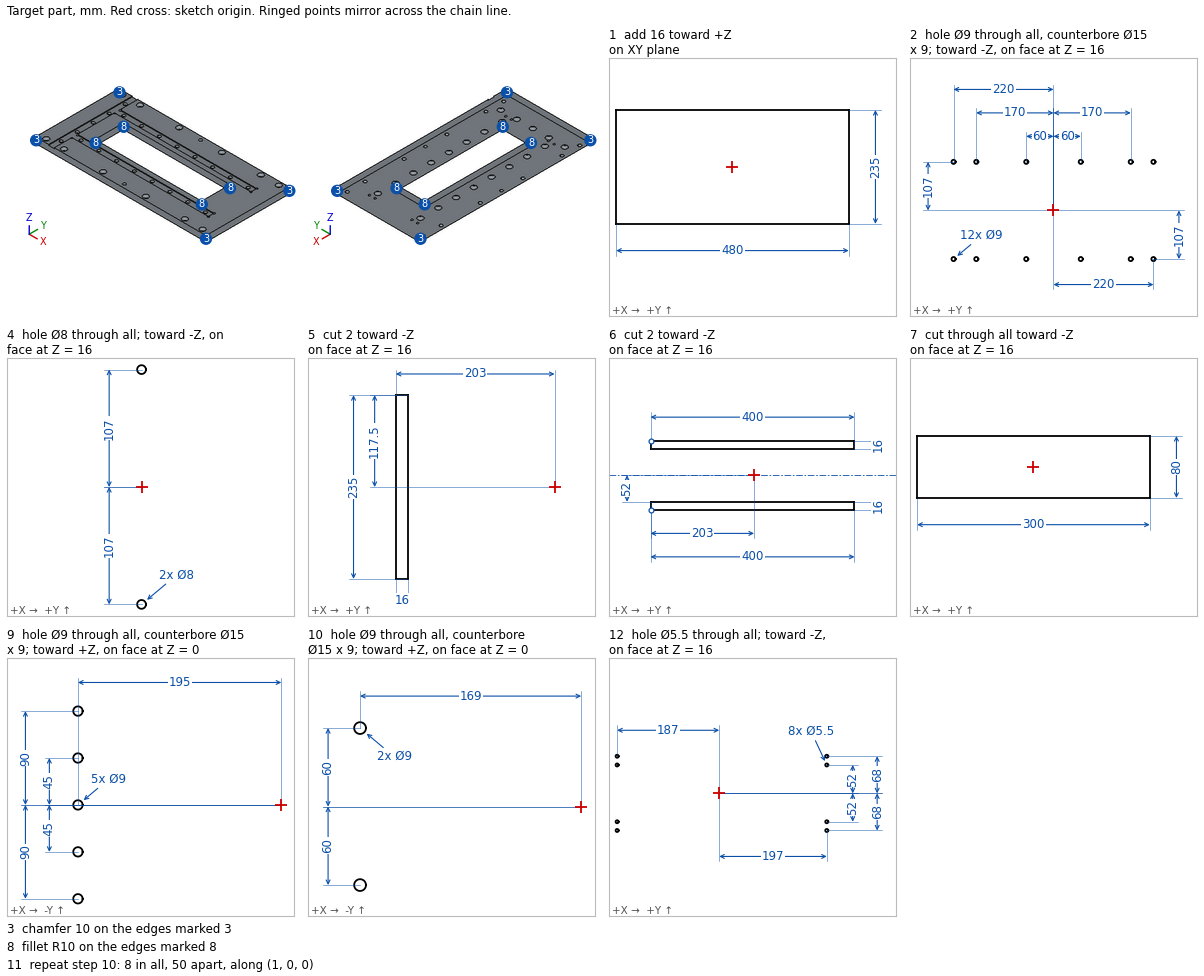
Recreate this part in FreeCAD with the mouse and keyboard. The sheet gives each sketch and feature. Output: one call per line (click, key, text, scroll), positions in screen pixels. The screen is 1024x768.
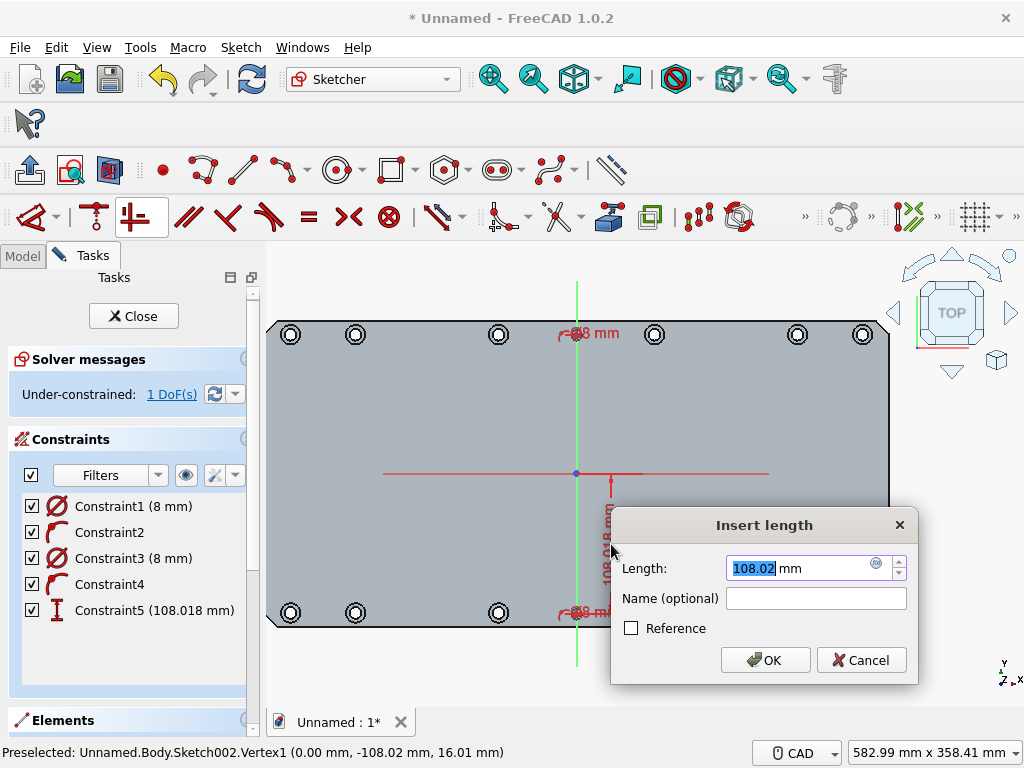
text(107)
key(Return)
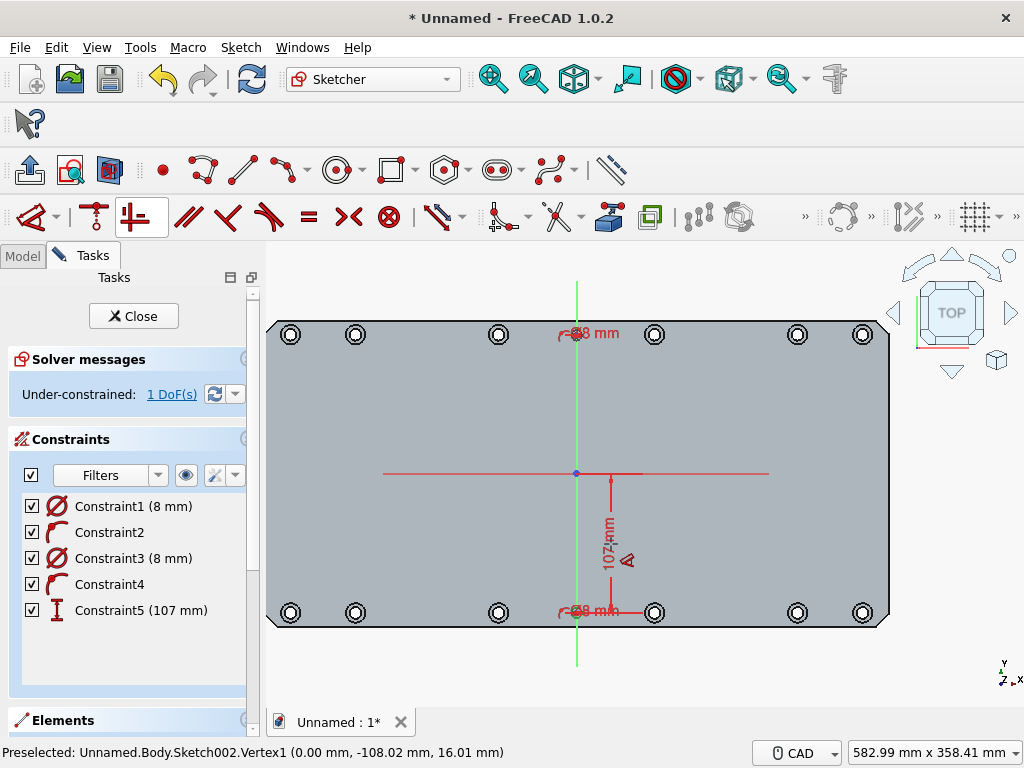
click(577, 335)
click(611, 405)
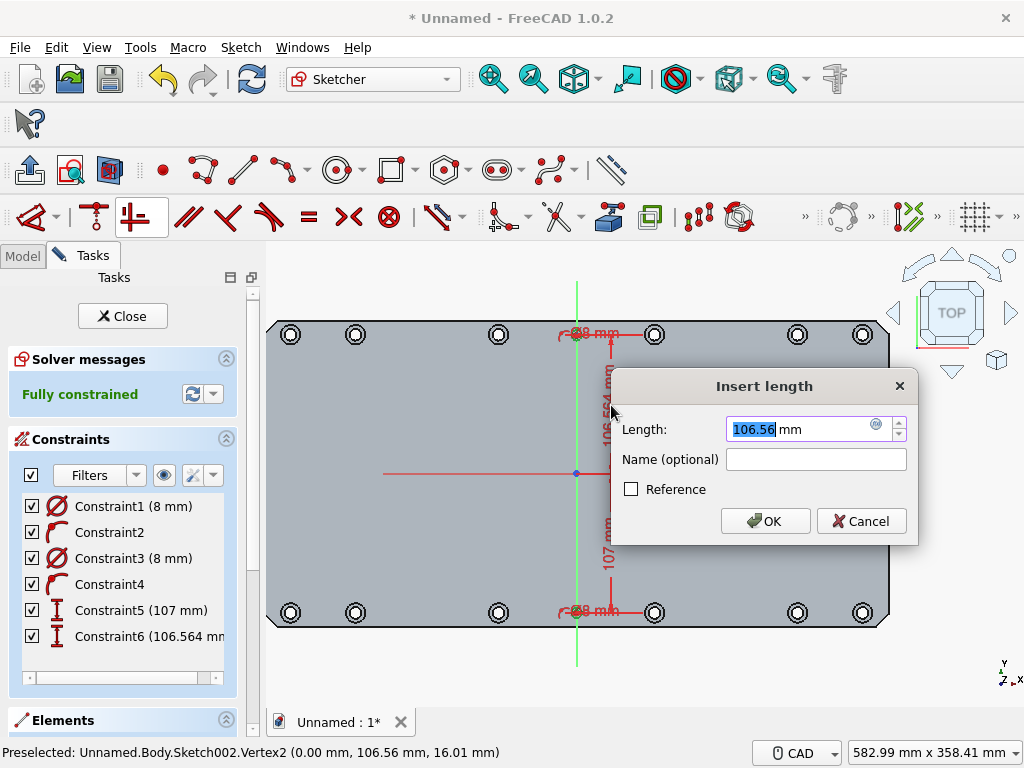
text(107)
key(Return)
key(Escape)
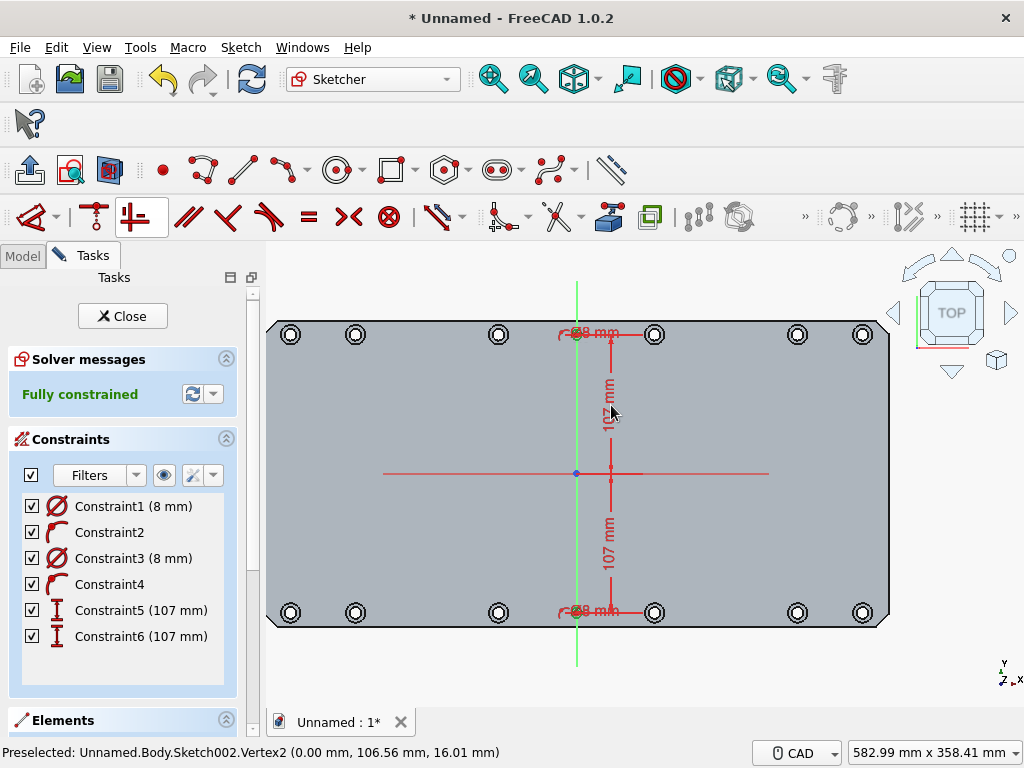
click(123, 316)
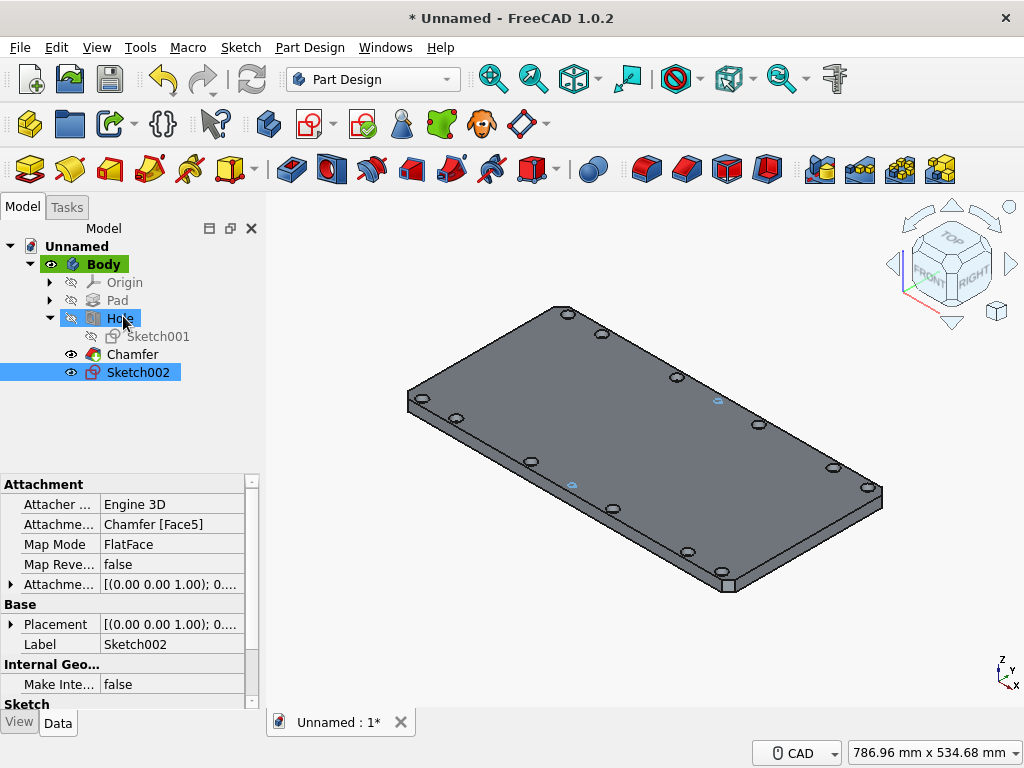
click(332, 170)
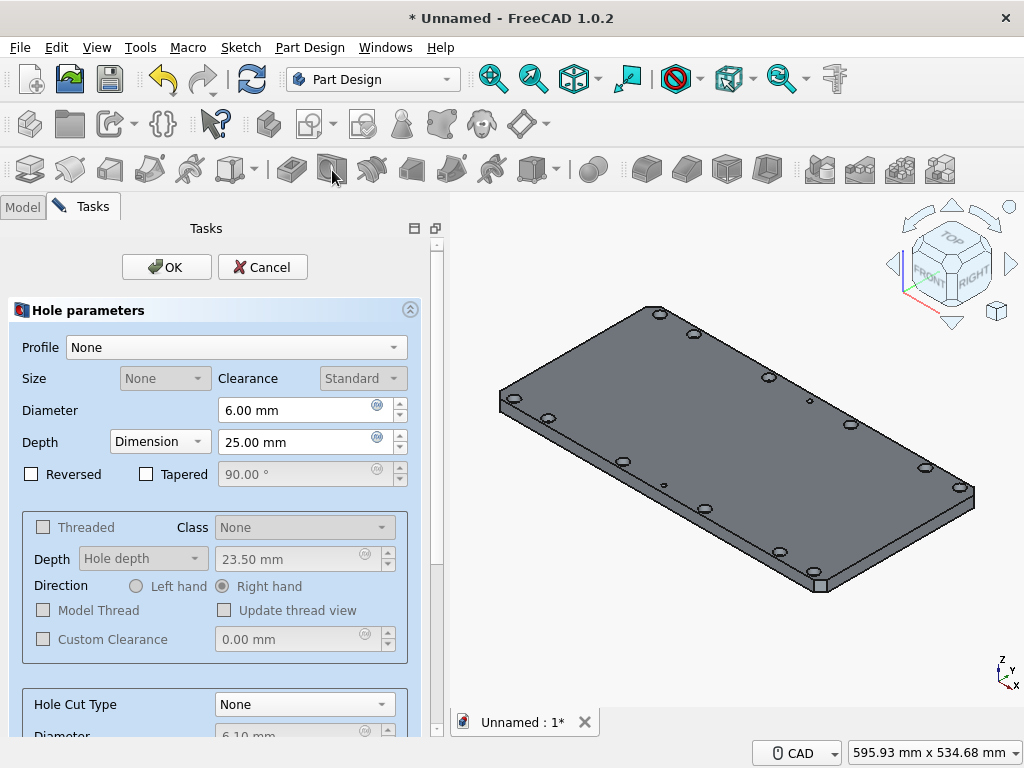
triple_click(305, 410)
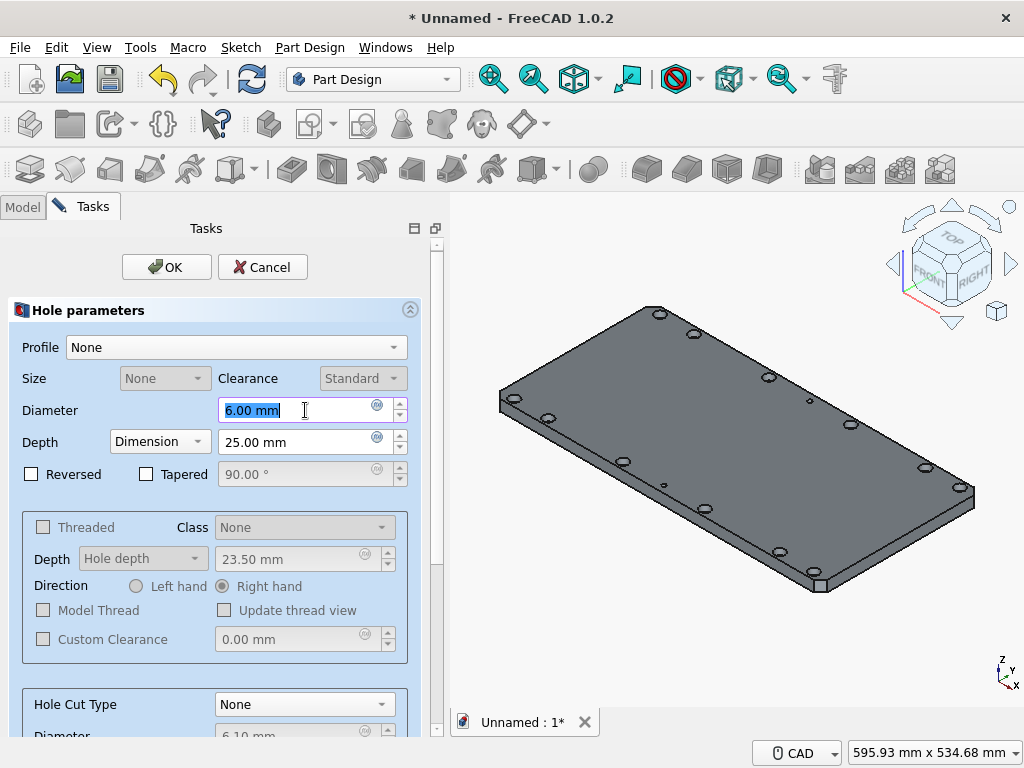
text(8)
key(Tab)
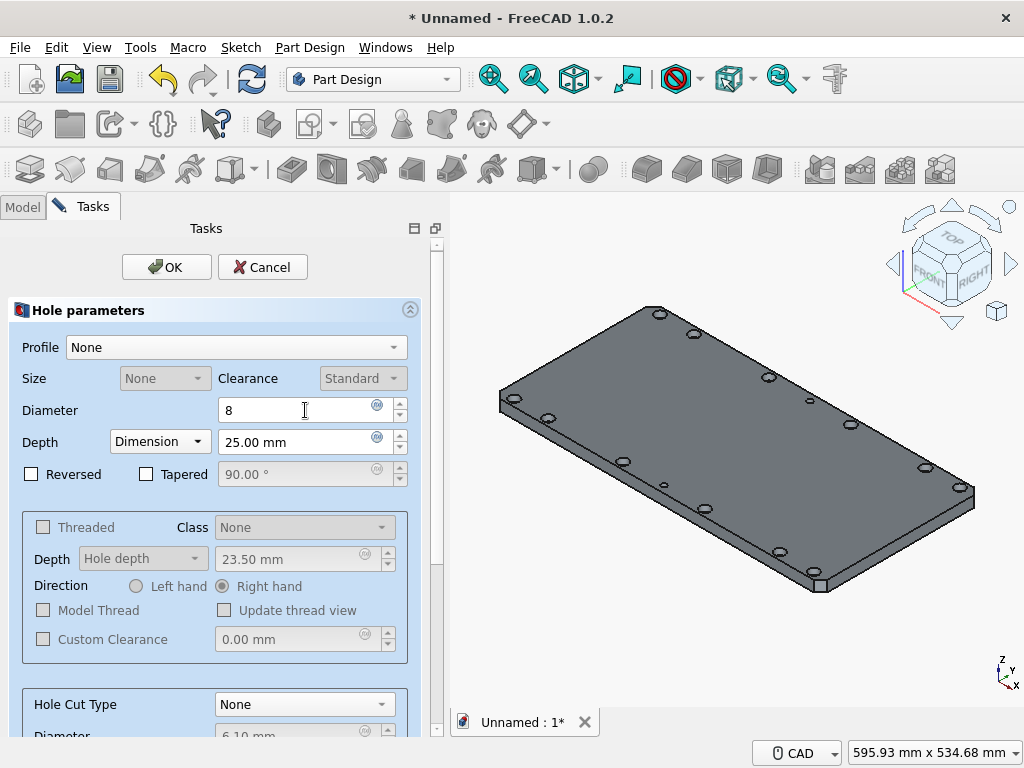
click(161, 442)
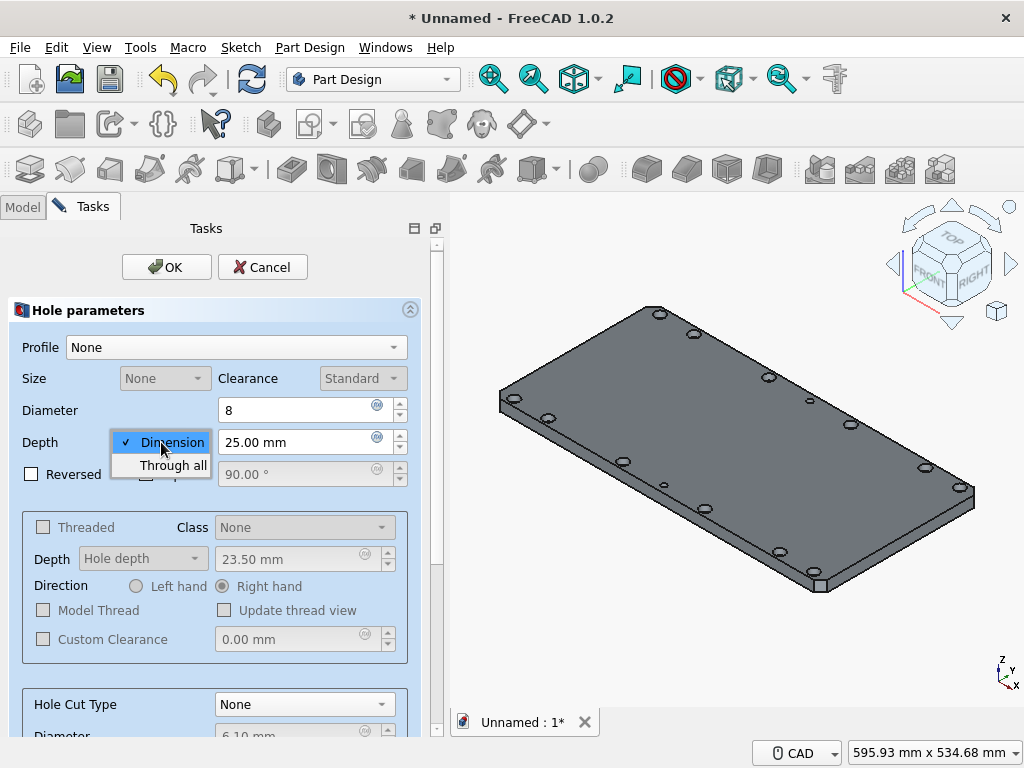
click(160, 466)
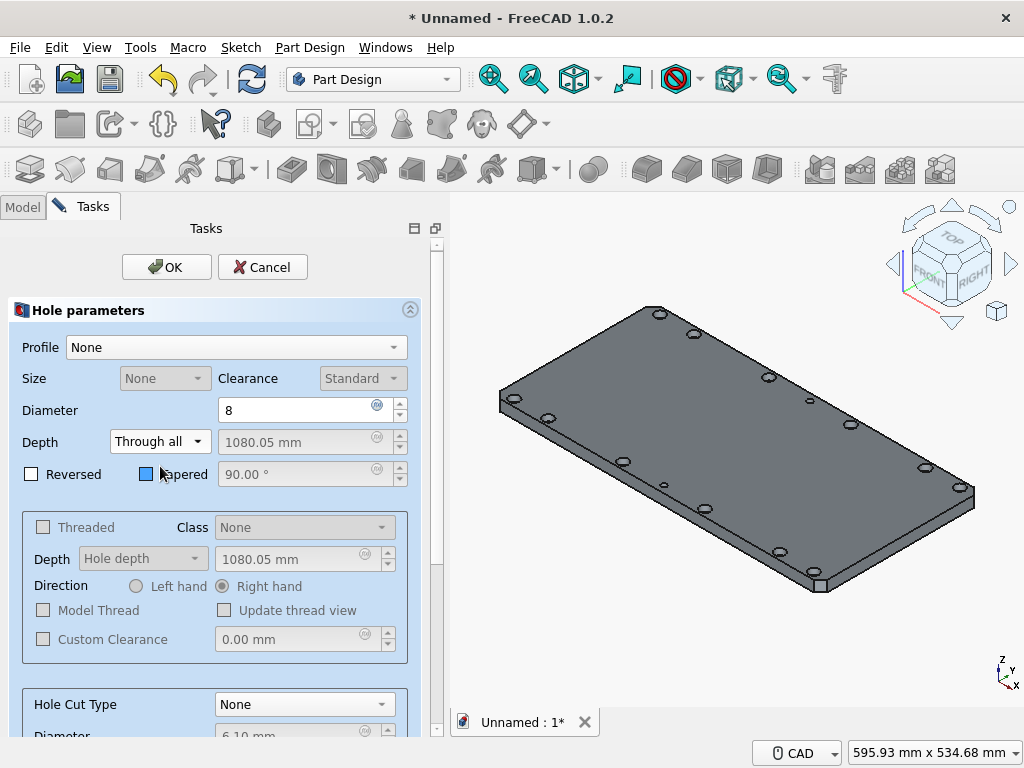
click(167, 267)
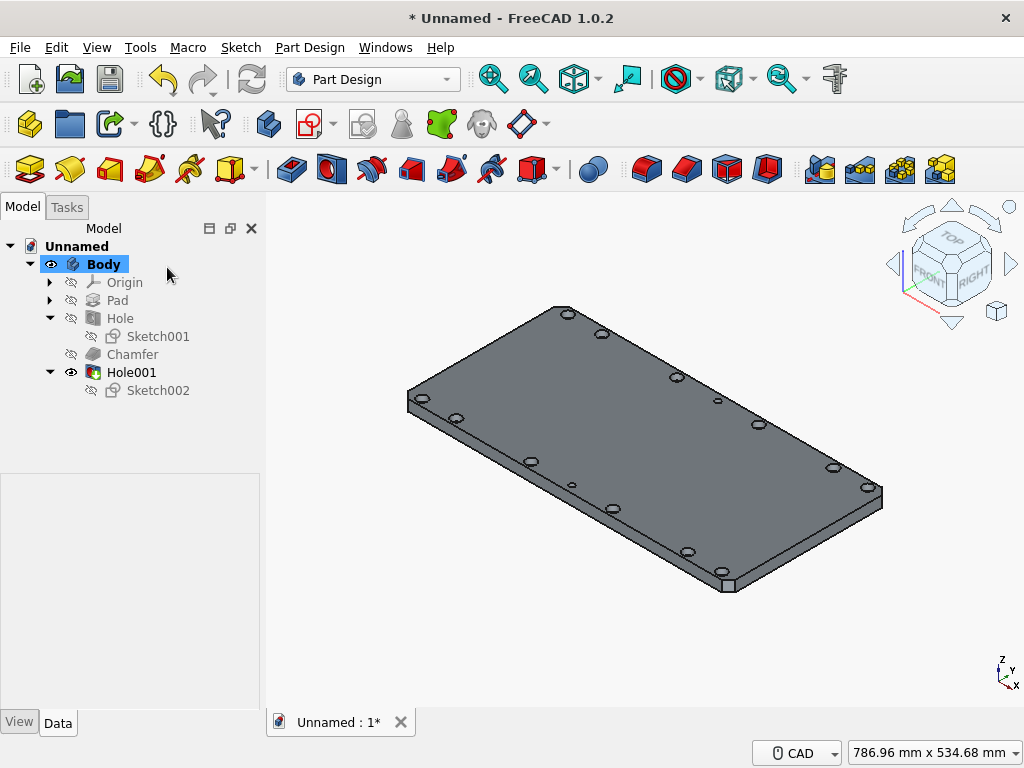
click(645, 442)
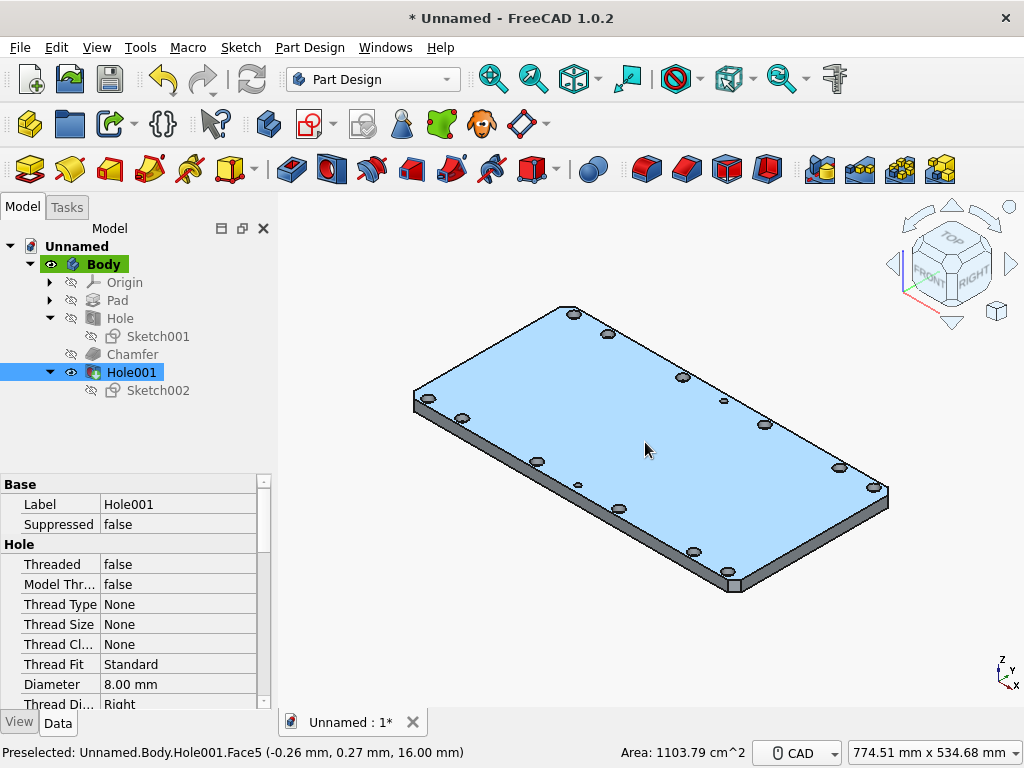
click(310, 124)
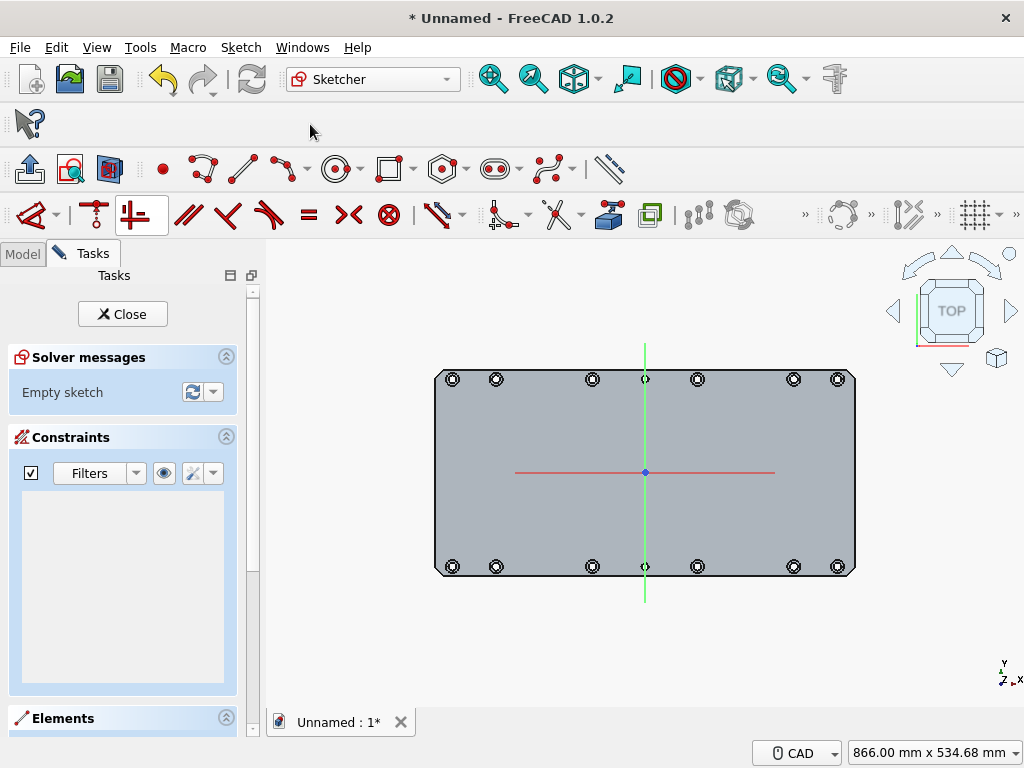
scroll(515, 473, up, 2)